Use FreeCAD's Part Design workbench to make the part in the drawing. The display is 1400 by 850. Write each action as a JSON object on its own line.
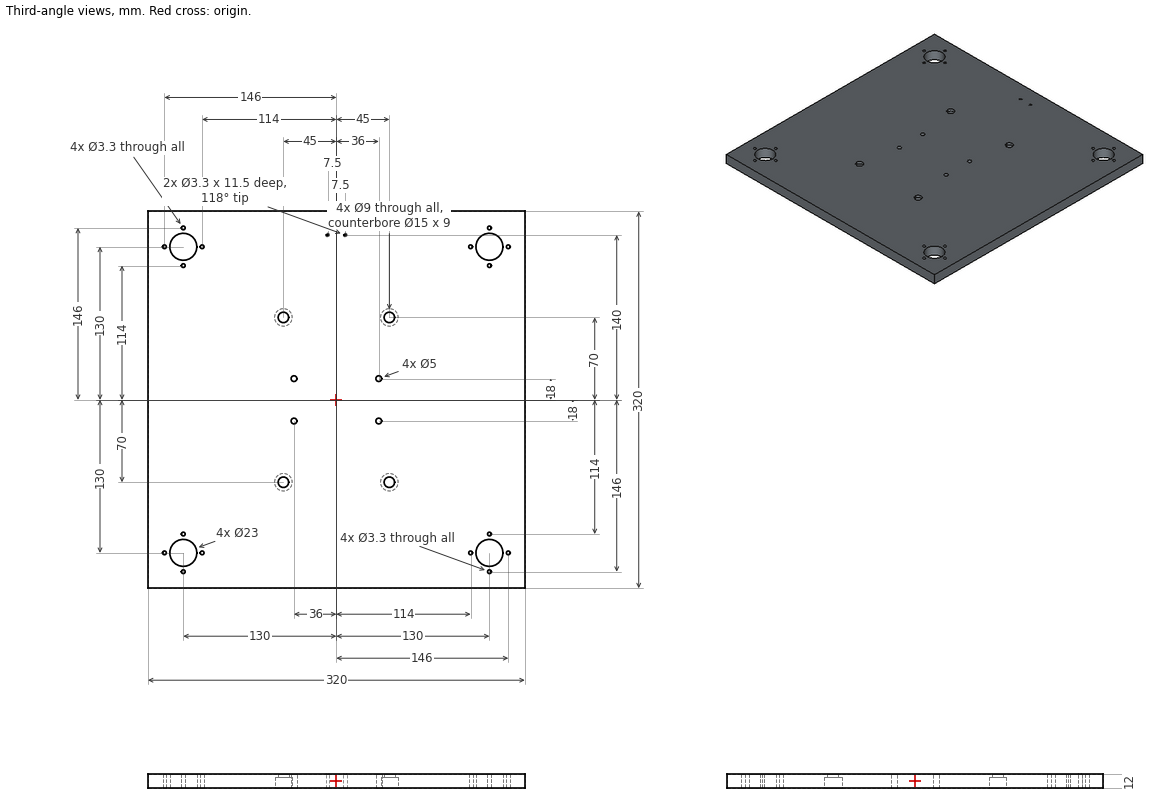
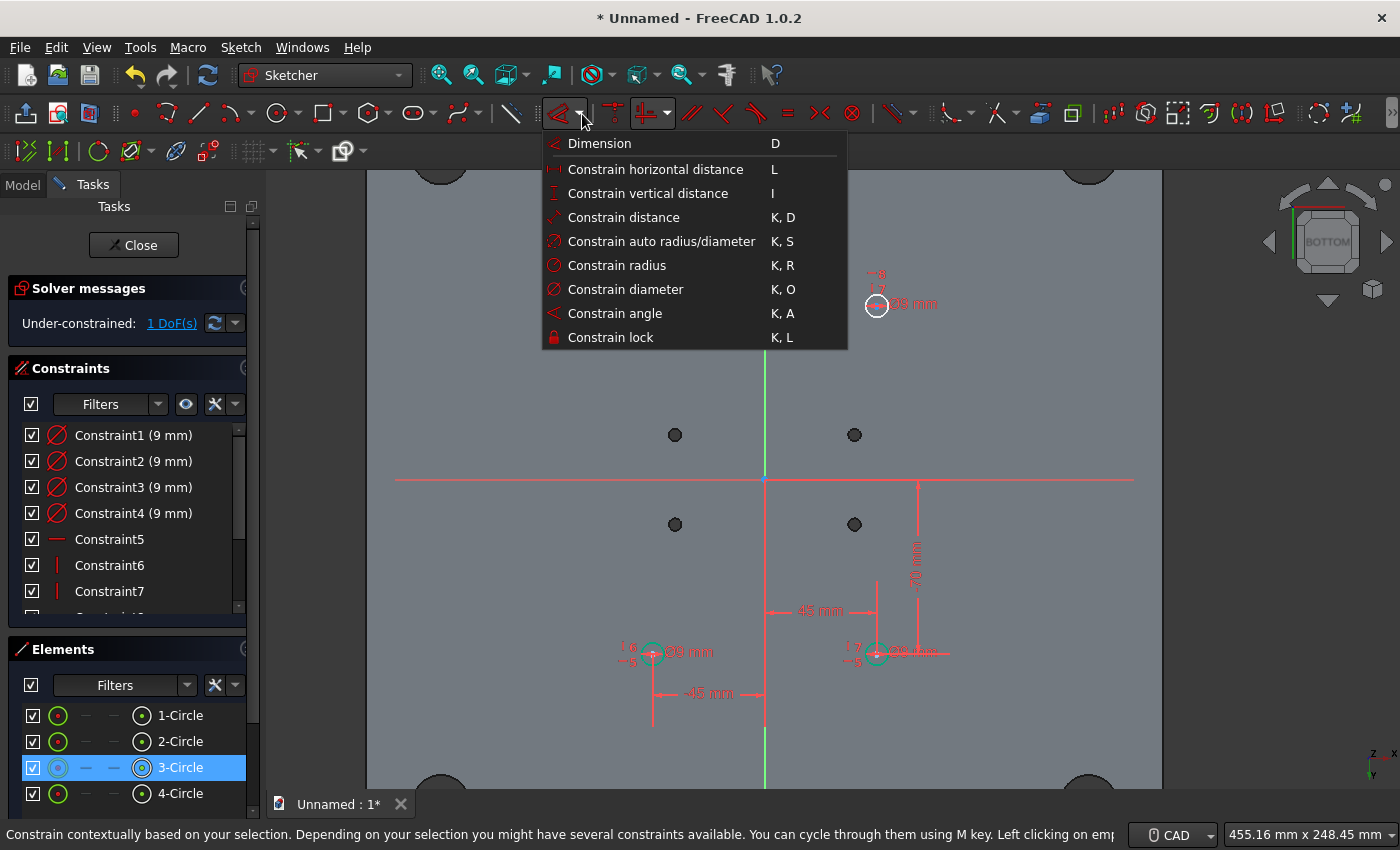
{"action": "left_click", "coordinate": [695, 193]}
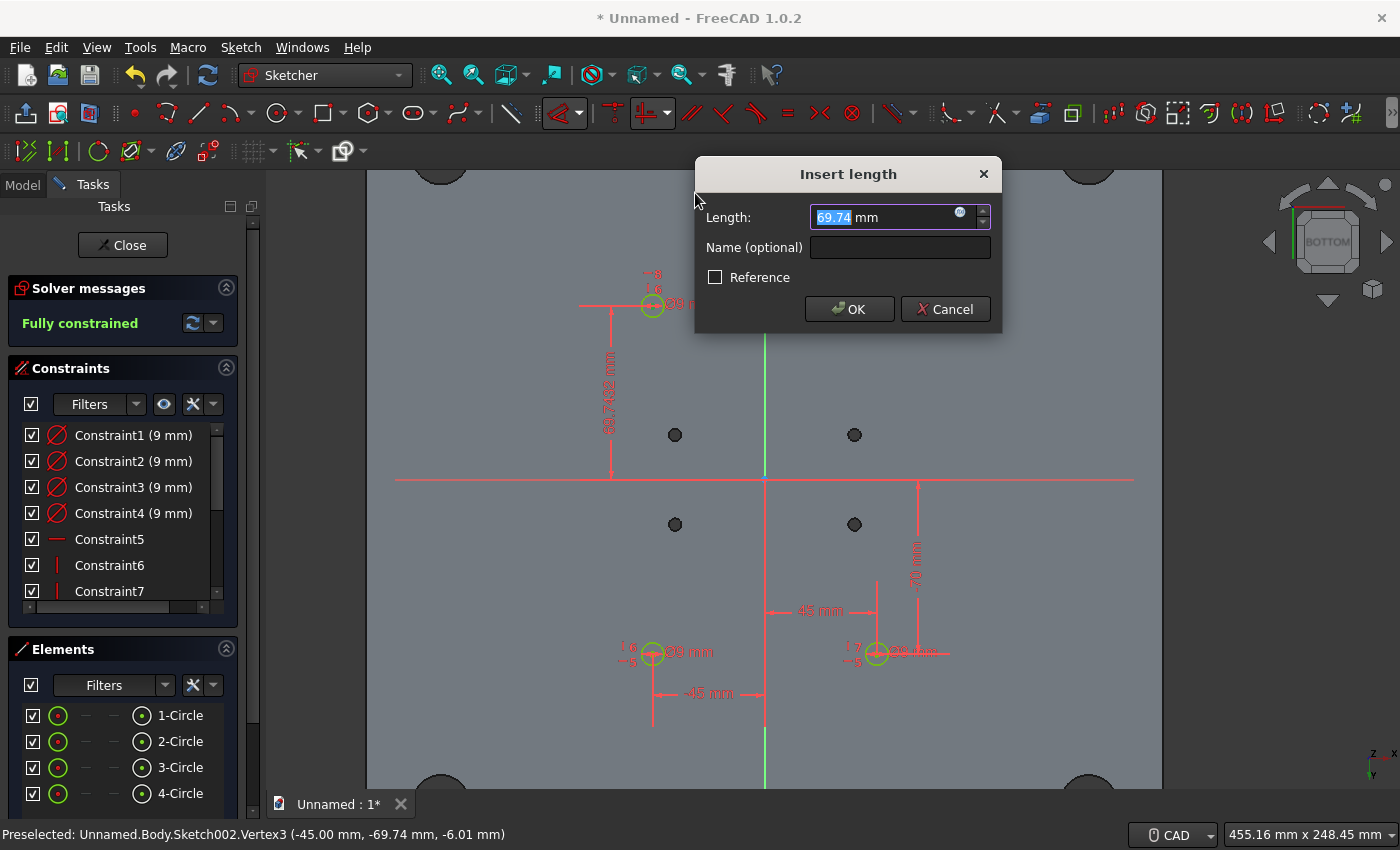
{"action": "type", "text": "70"}
{"action": "key", "text": "Return"}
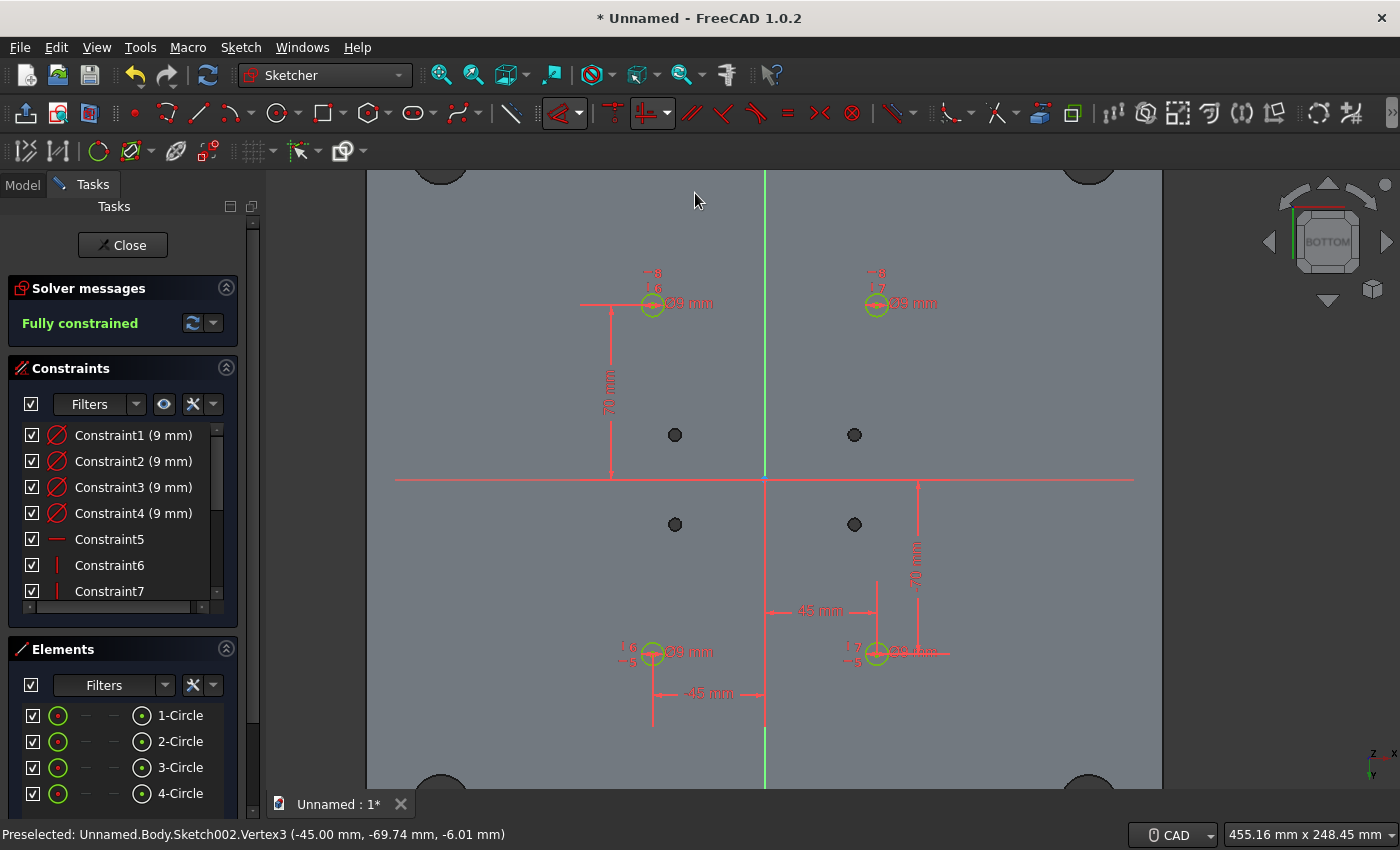
{"action": "left_click", "coordinate": [123, 245]}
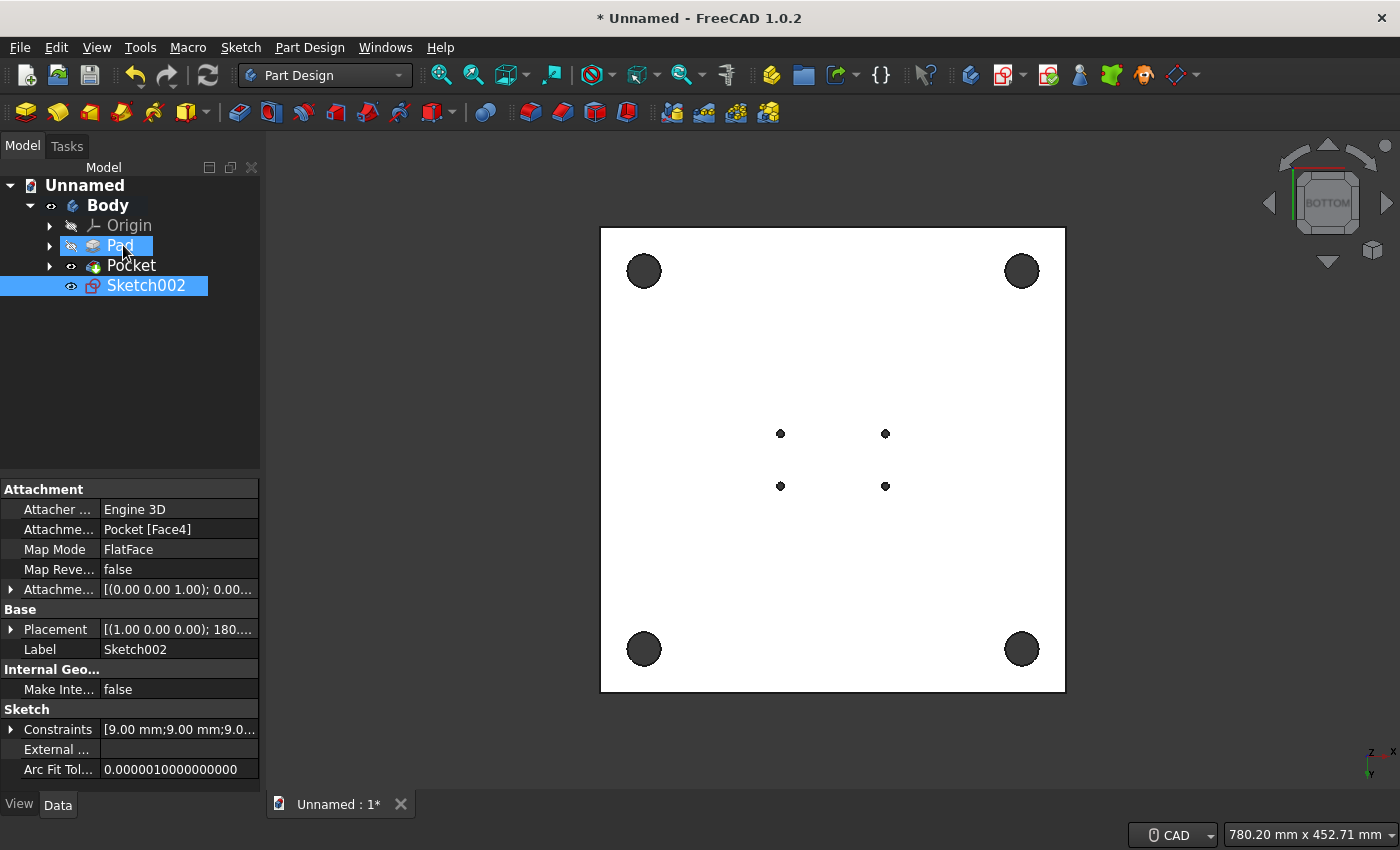
{"action": "left_click", "coordinate": [272, 112]}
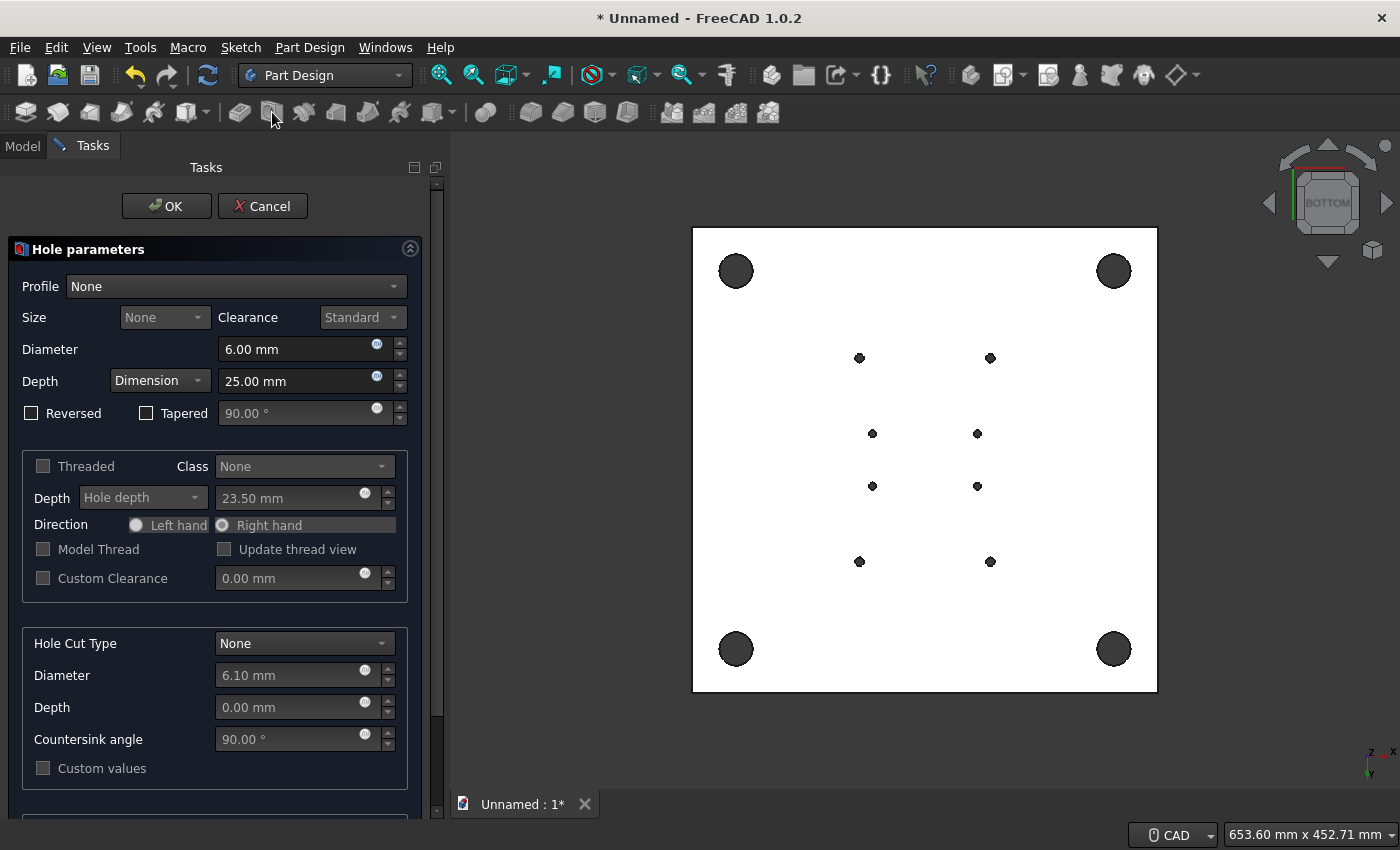
{"action": "triple_click", "coordinate": [305, 349]}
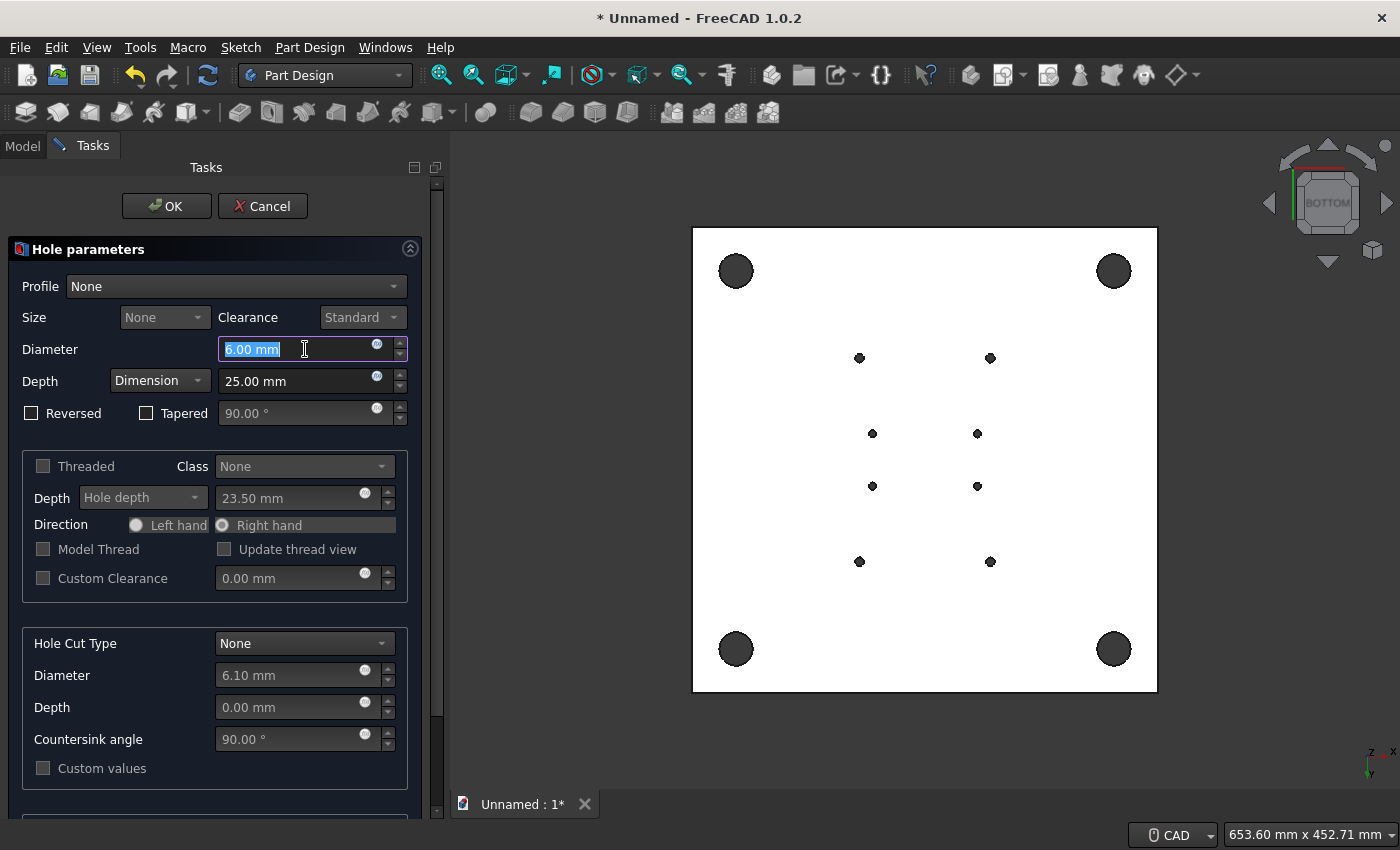
{"action": "type", "text": "9"}
{"action": "key", "text": "Tab"}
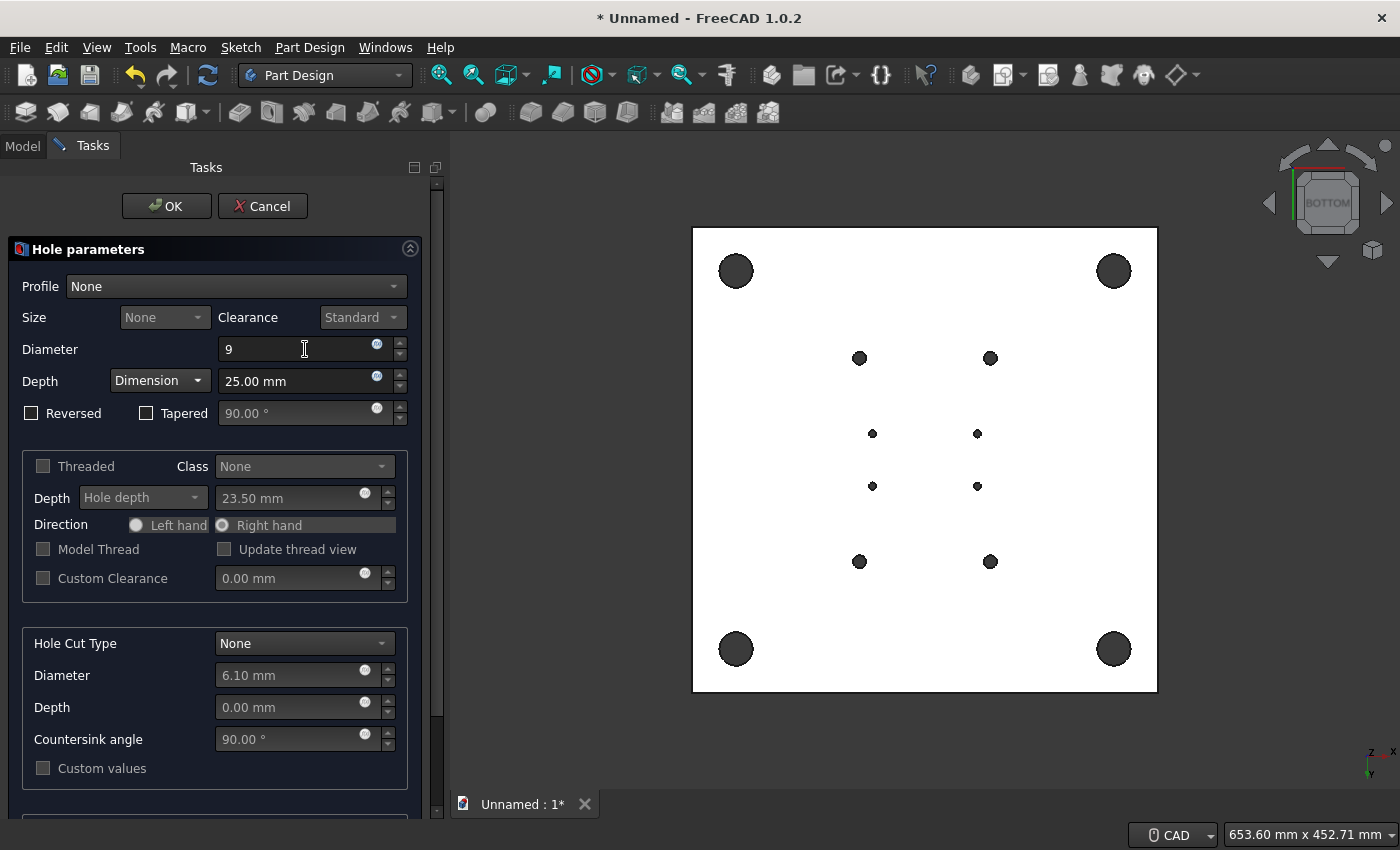
{"action": "left_click", "coordinate": [161, 380]}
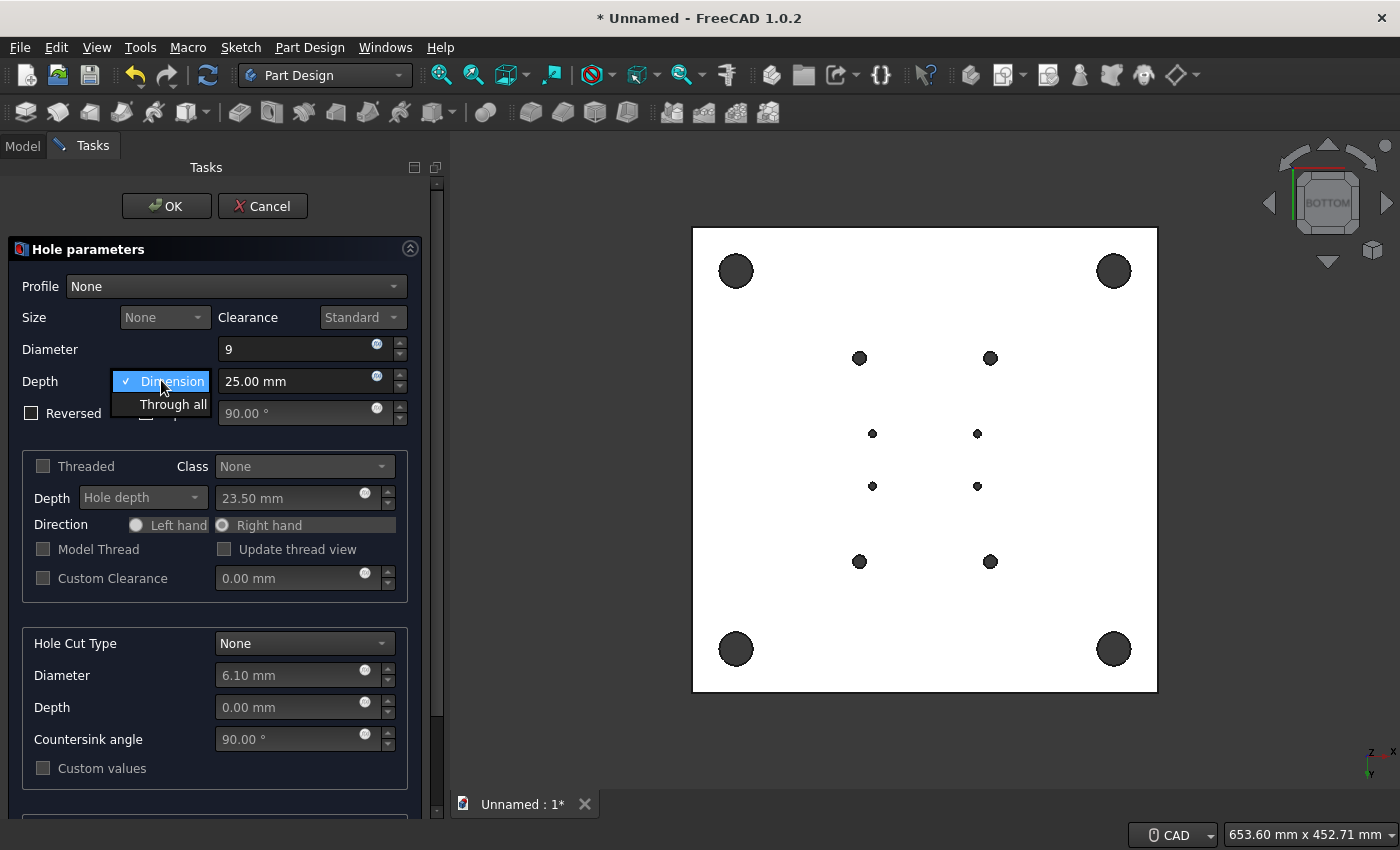
{"action": "left_click", "coordinate": [160, 404]}